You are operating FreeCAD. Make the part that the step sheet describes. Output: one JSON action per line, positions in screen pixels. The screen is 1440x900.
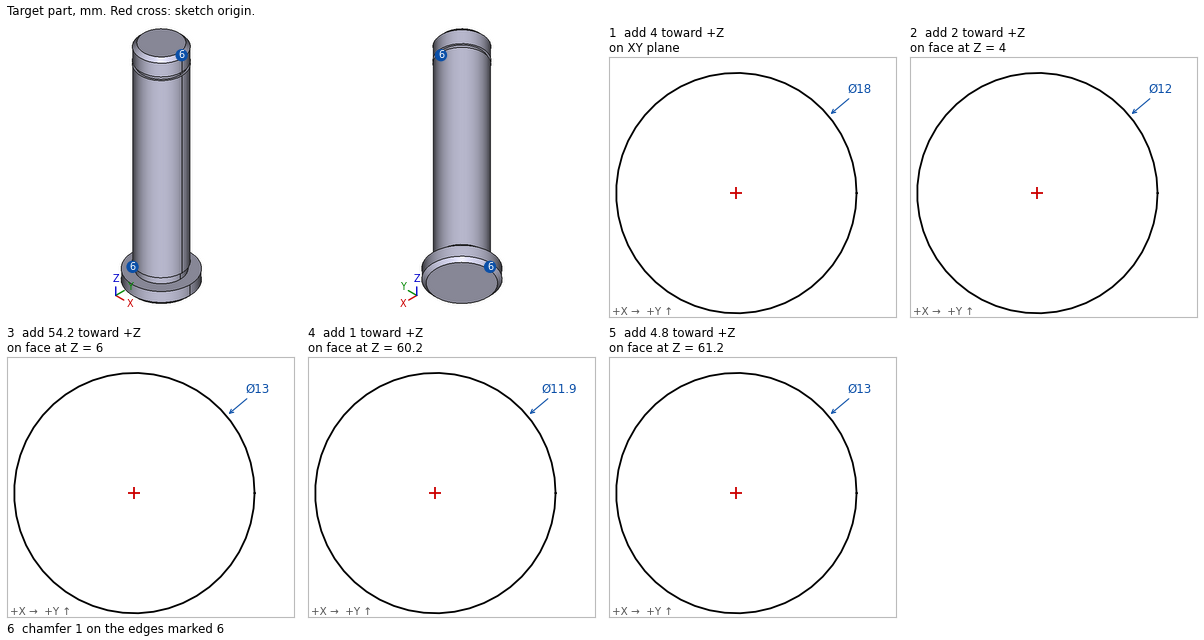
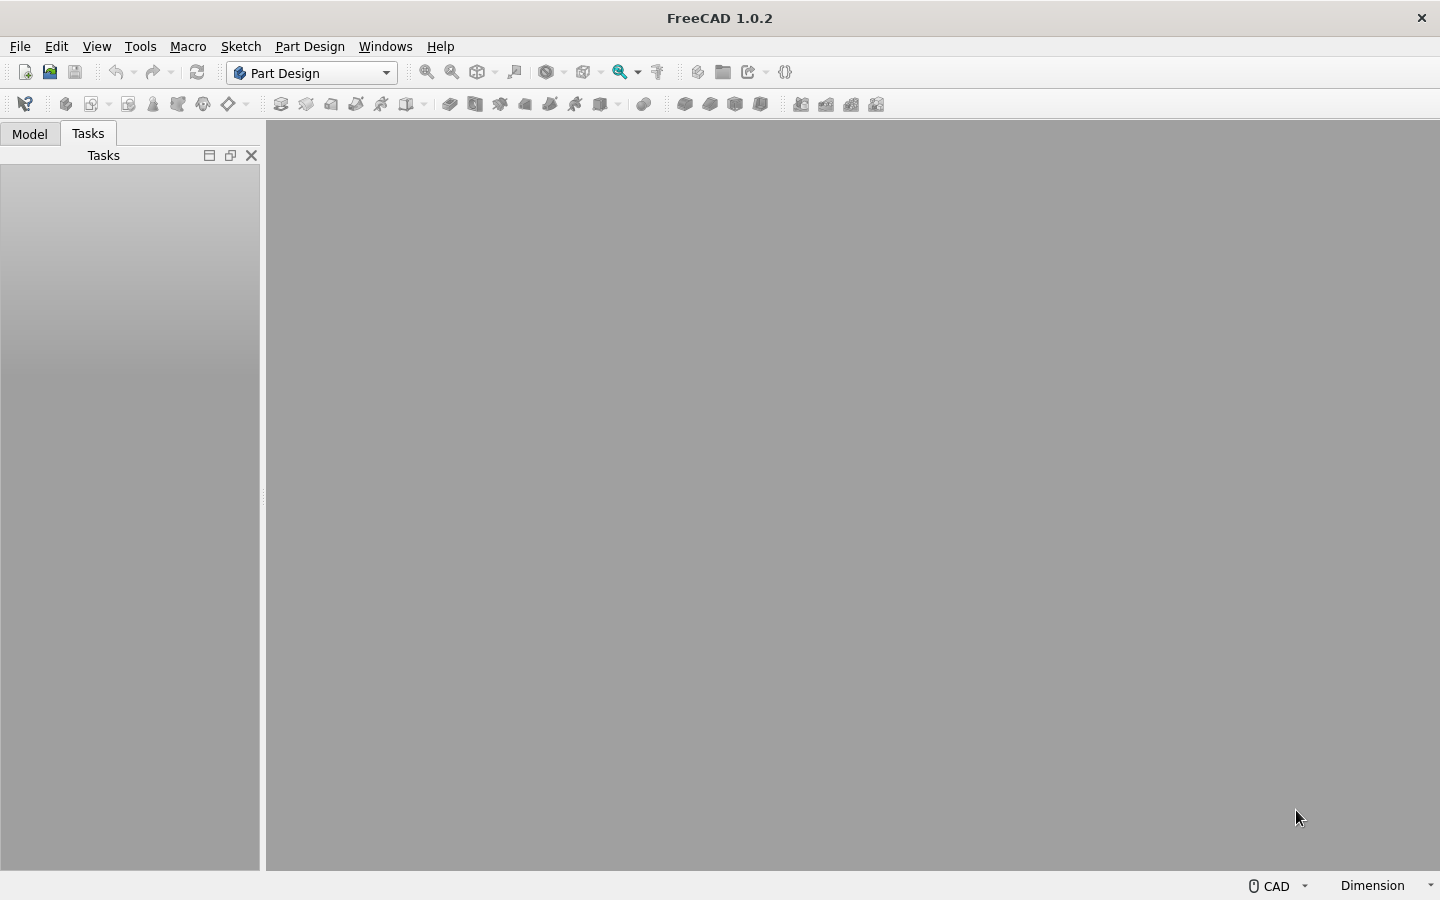
{"action": "left_click", "coordinate": [25, 72]}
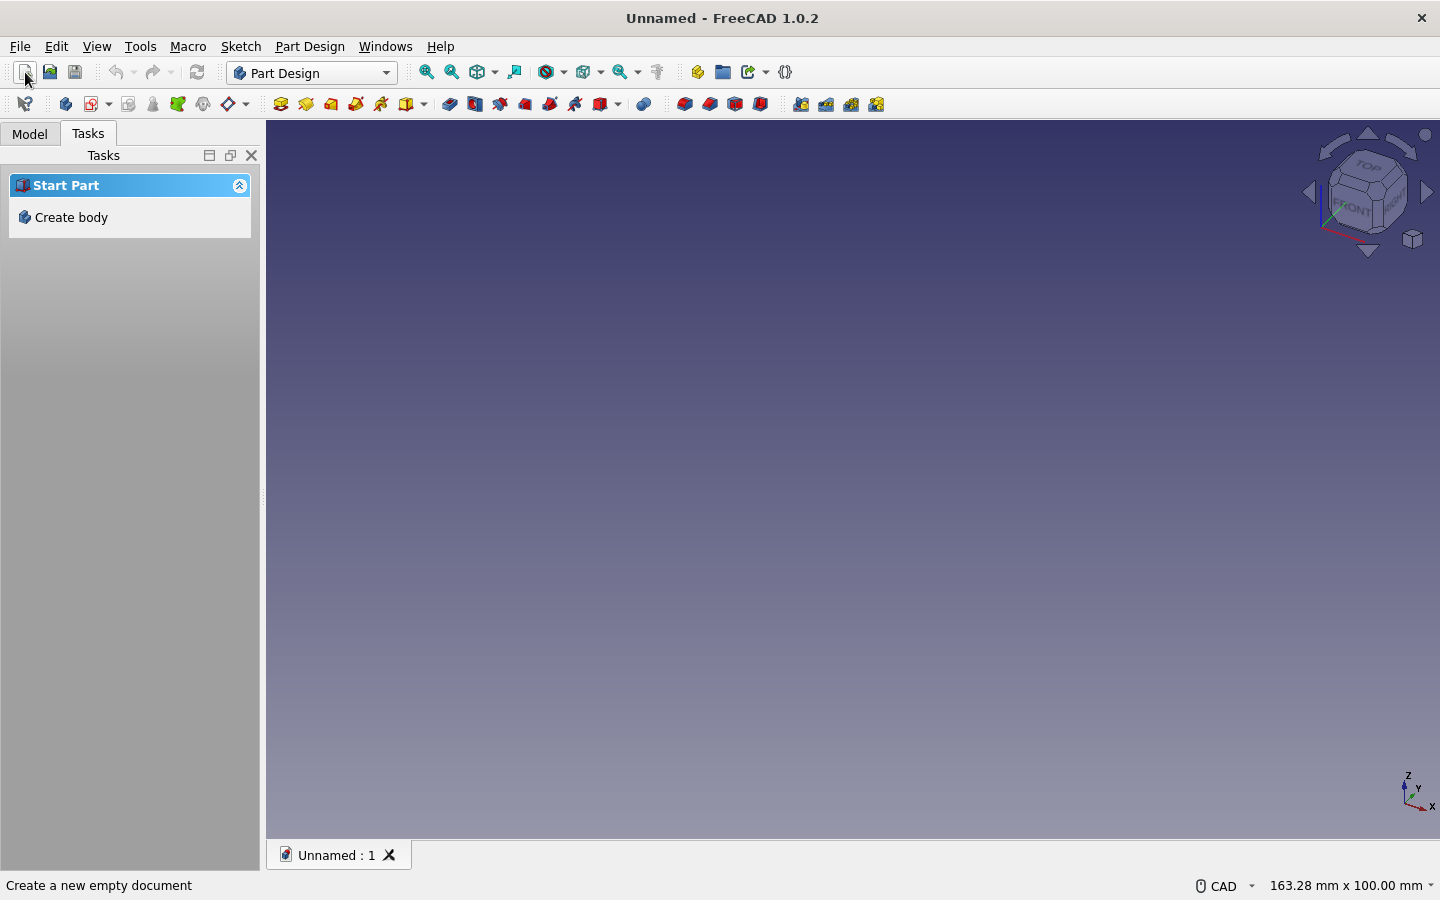
{"action": "left_click", "coordinate": [90, 104]}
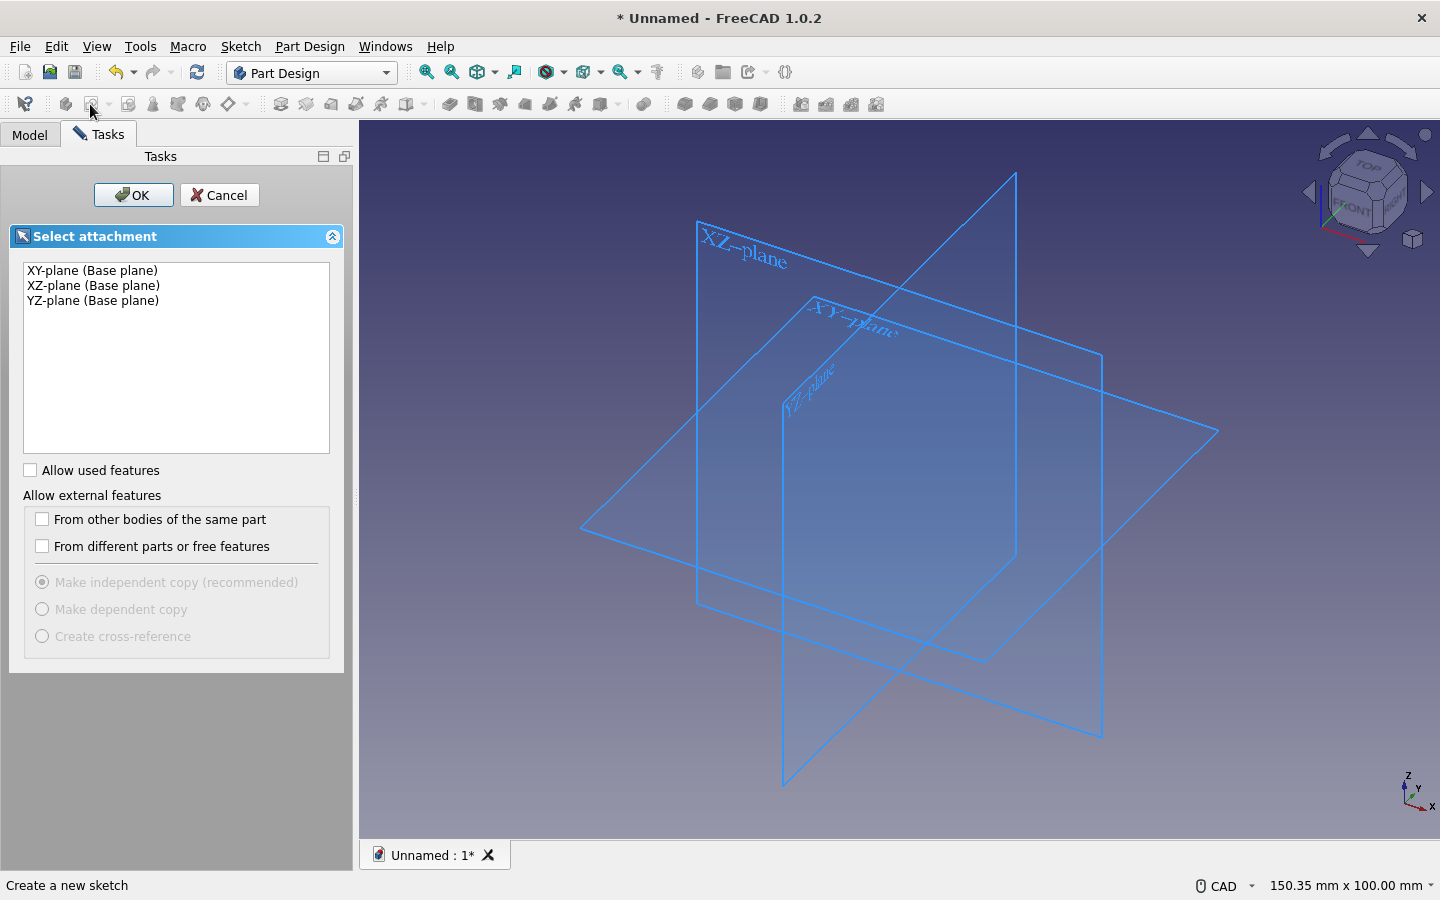
{"action": "left_click", "coordinate": [84, 270]}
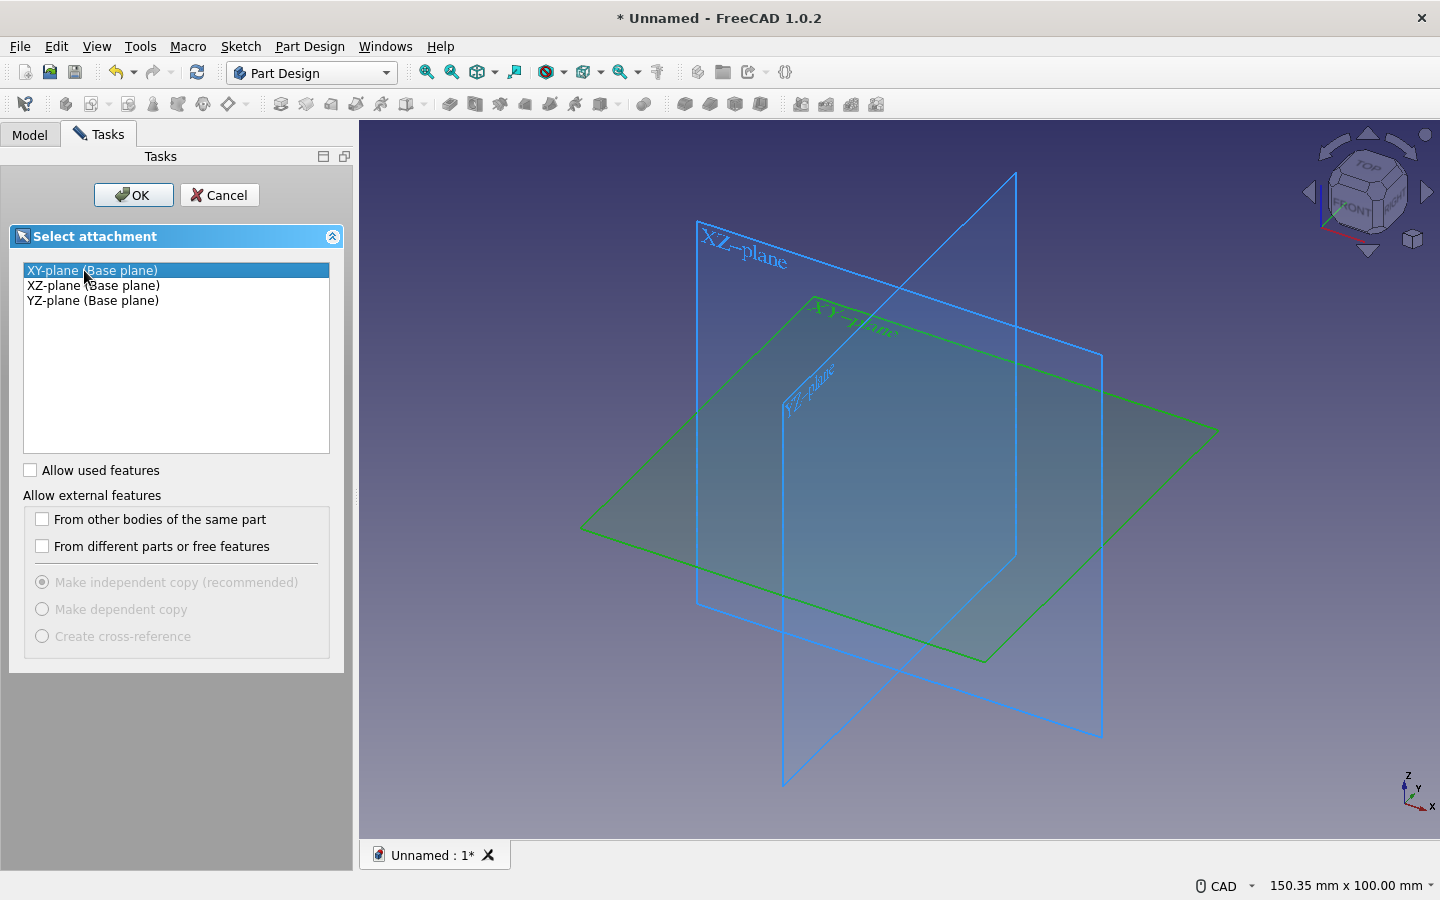
{"action": "left_click", "coordinate": [134, 195]}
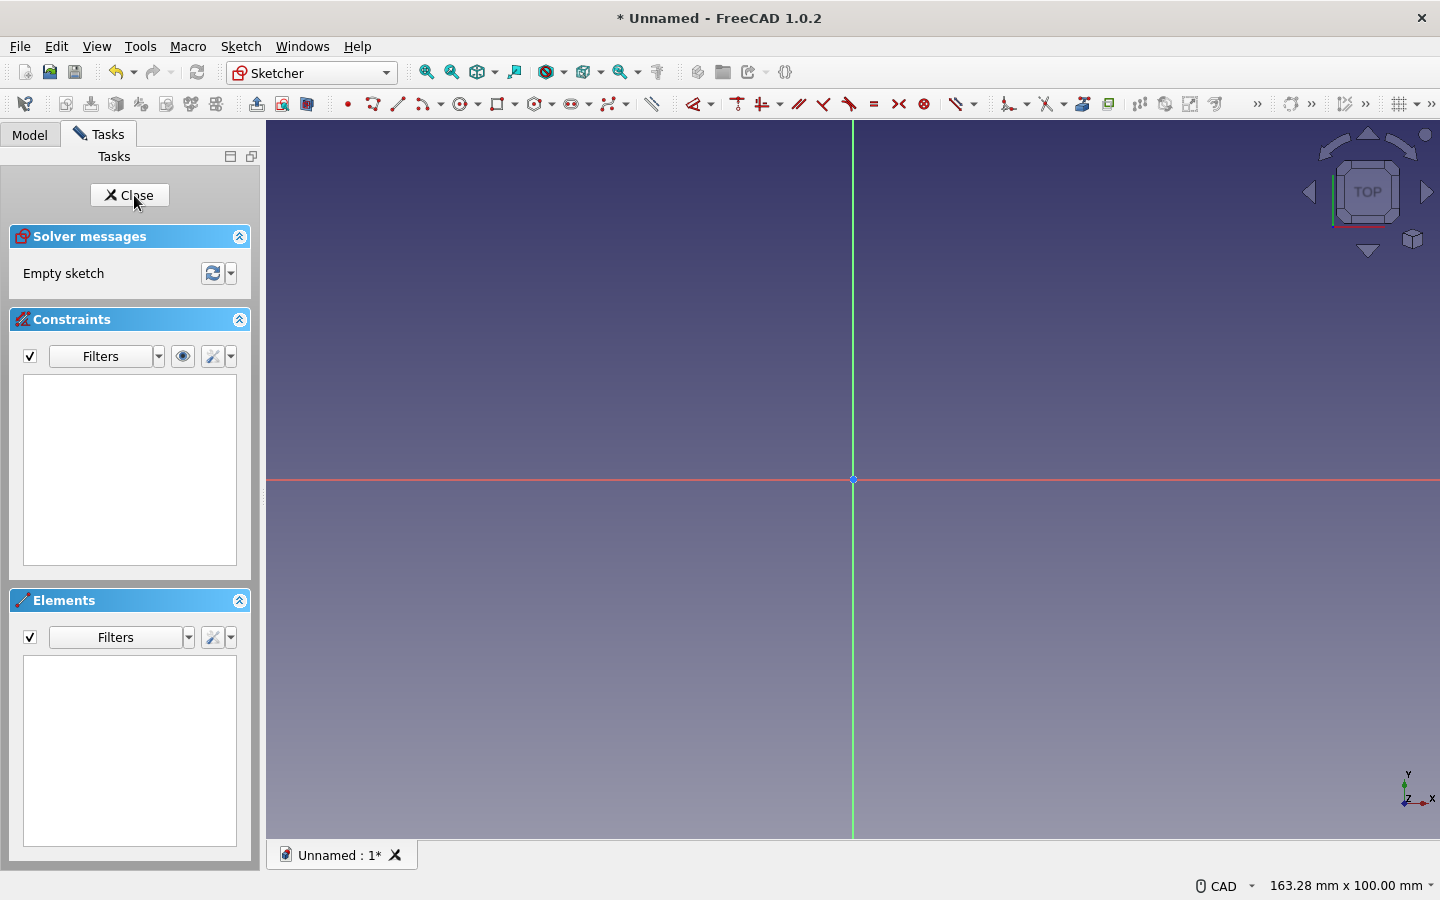
{"action": "scroll", "coordinate": [883, 480], "scroll_direction": "up", "scroll_amount": 6}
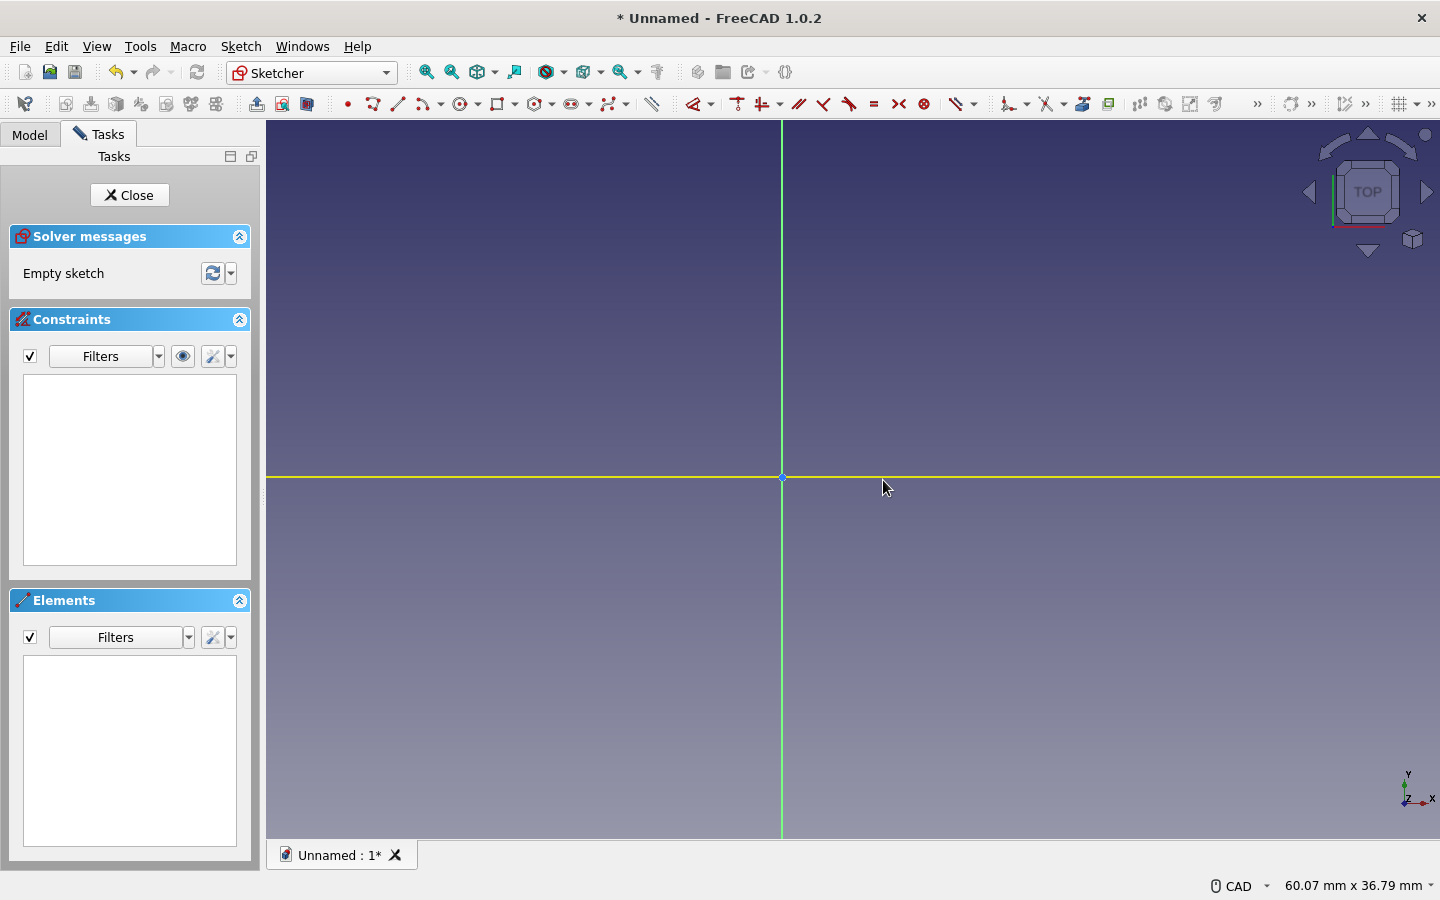
{"action": "left_click", "coordinate": [460, 104]}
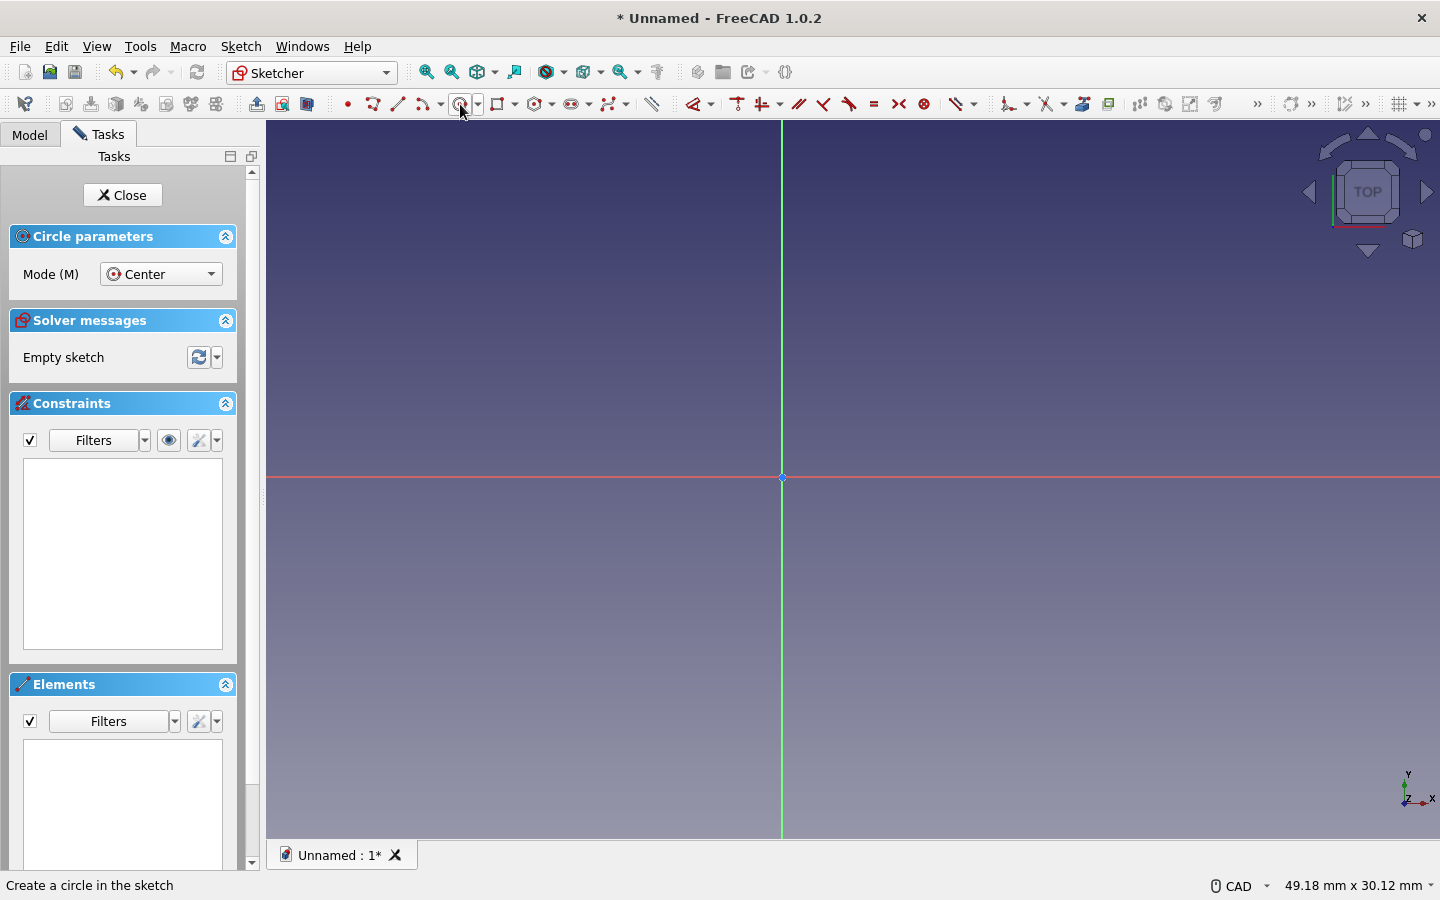
{"action": "left_click", "coordinate": [782, 477]}
{"action": "left_click", "coordinate": [934, 325]}
{"action": "key", "text": "Escape"}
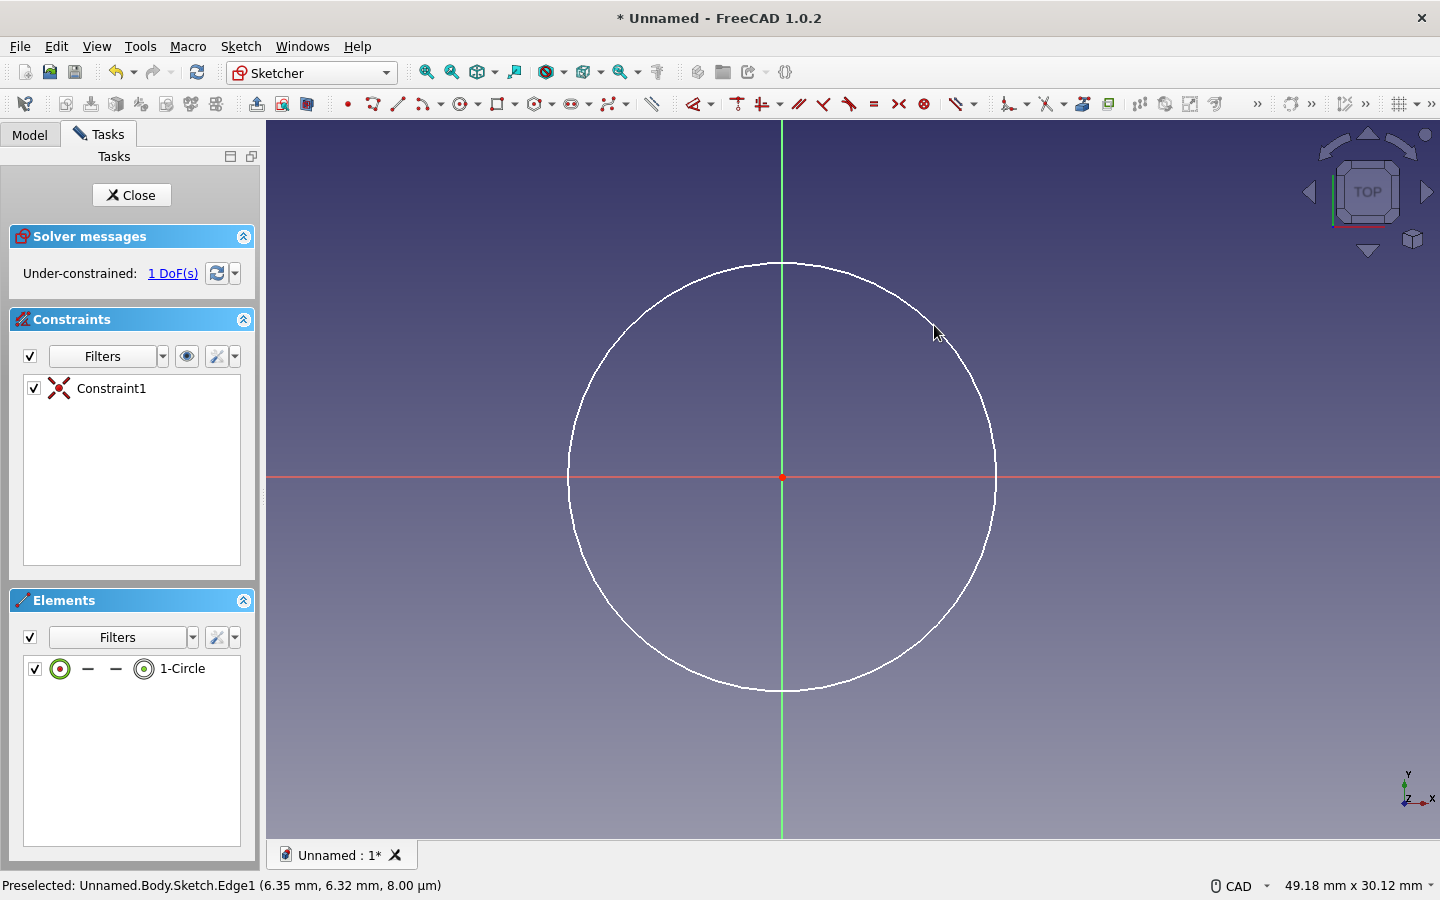
{"action": "left_click", "coordinate": [692, 104]}